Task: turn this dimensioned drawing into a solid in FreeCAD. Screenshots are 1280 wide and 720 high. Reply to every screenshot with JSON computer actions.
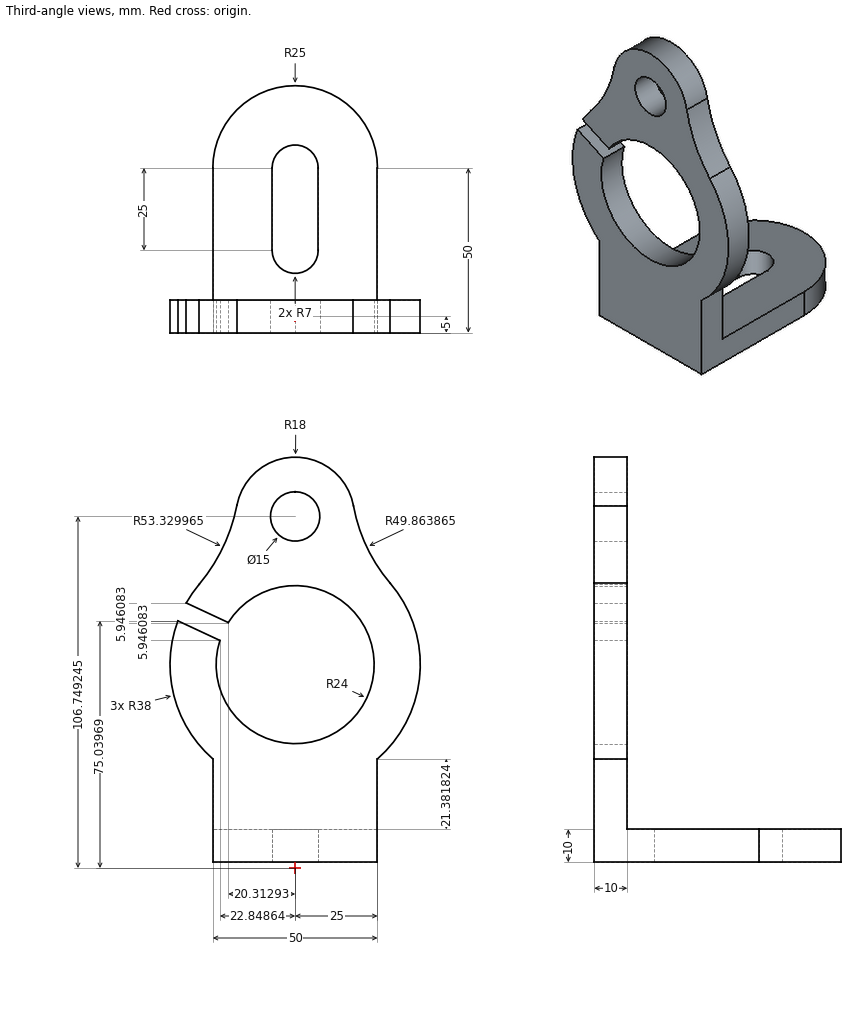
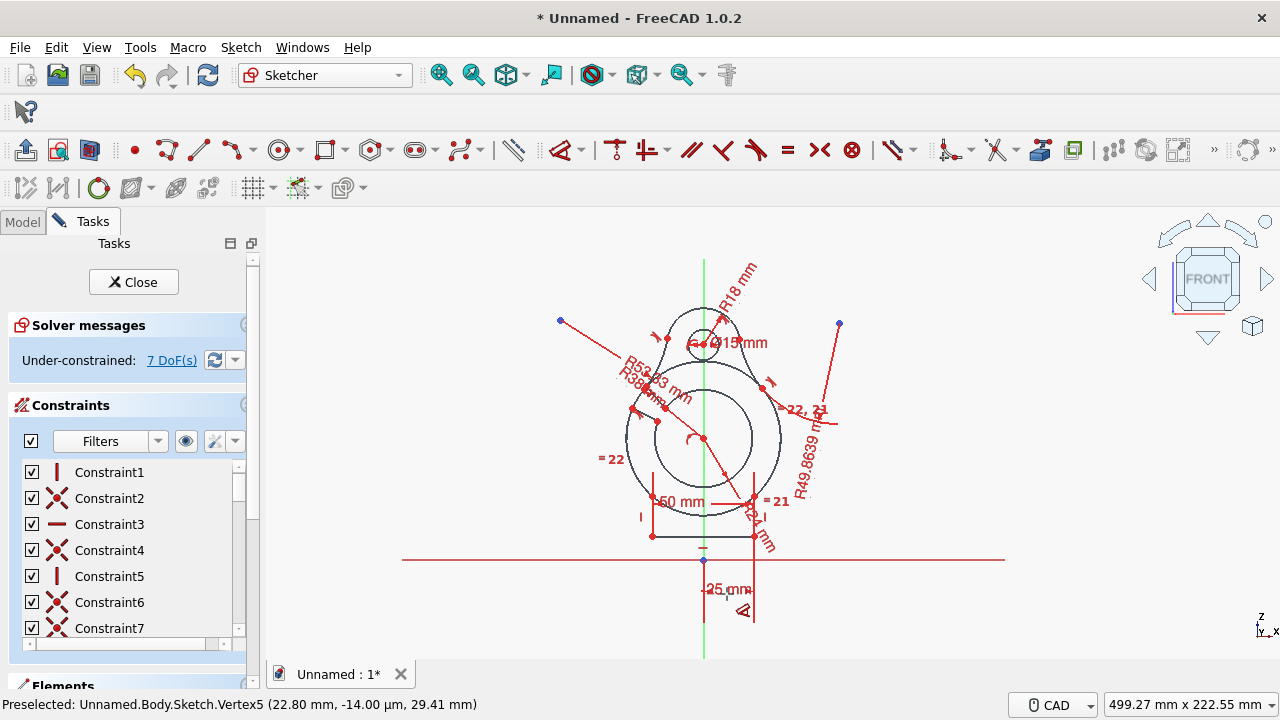
{"action": "scroll", "coordinate": [754, 509], "scroll_direction": "up", "scroll_amount": 2}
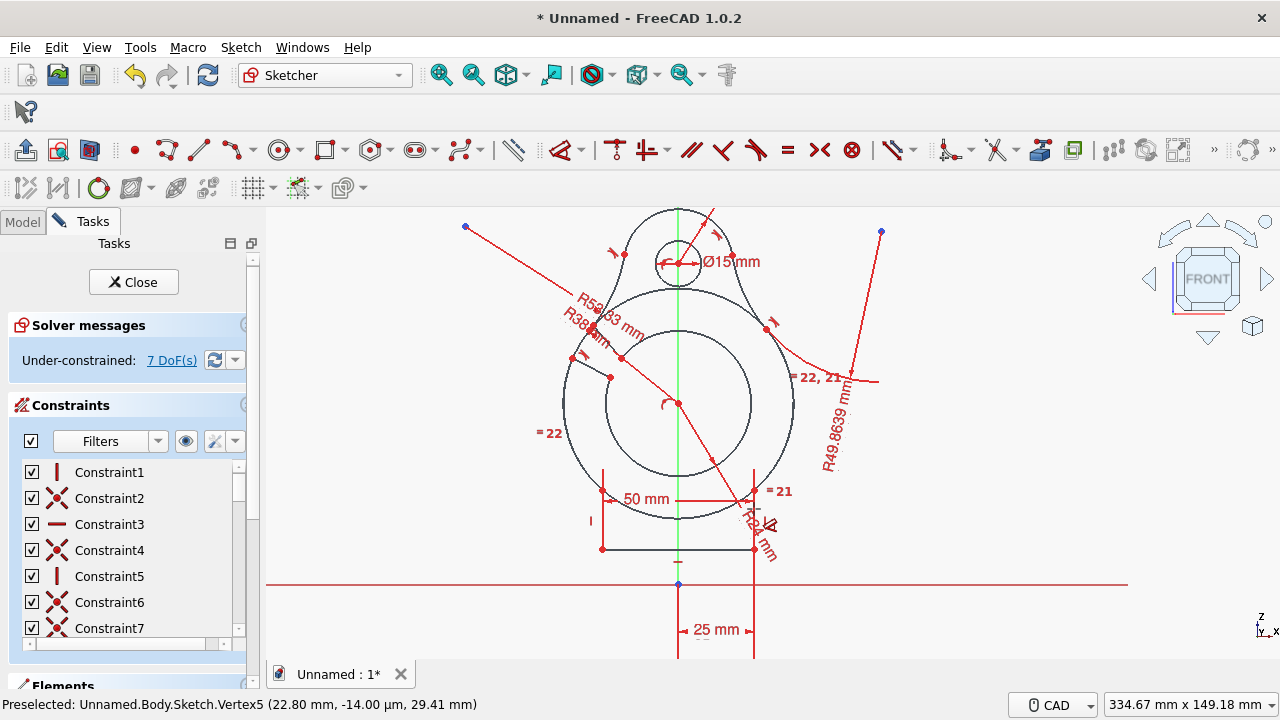
{"action": "left_click", "coordinate": [754, 508]}
{"action": "left_click", "coordinate": [788, 506]}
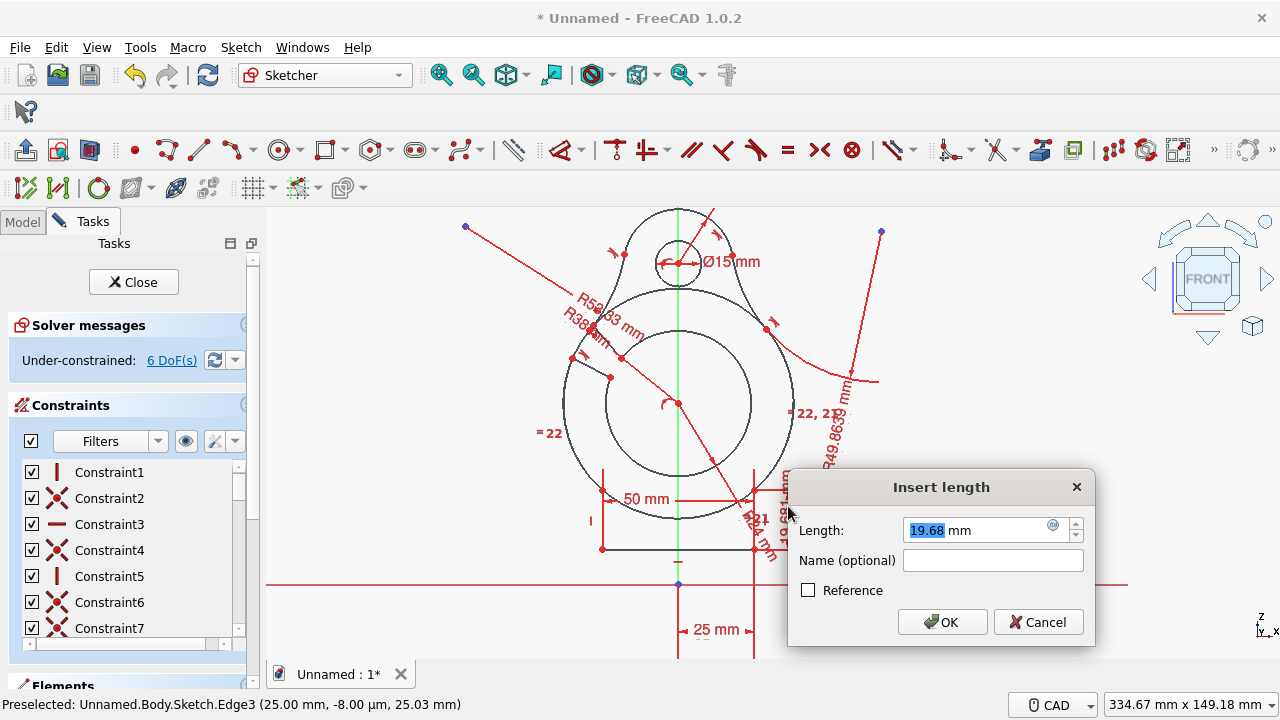
{"action": "type", "text": "21.381824"}
{"action": "key", "text": "Return"}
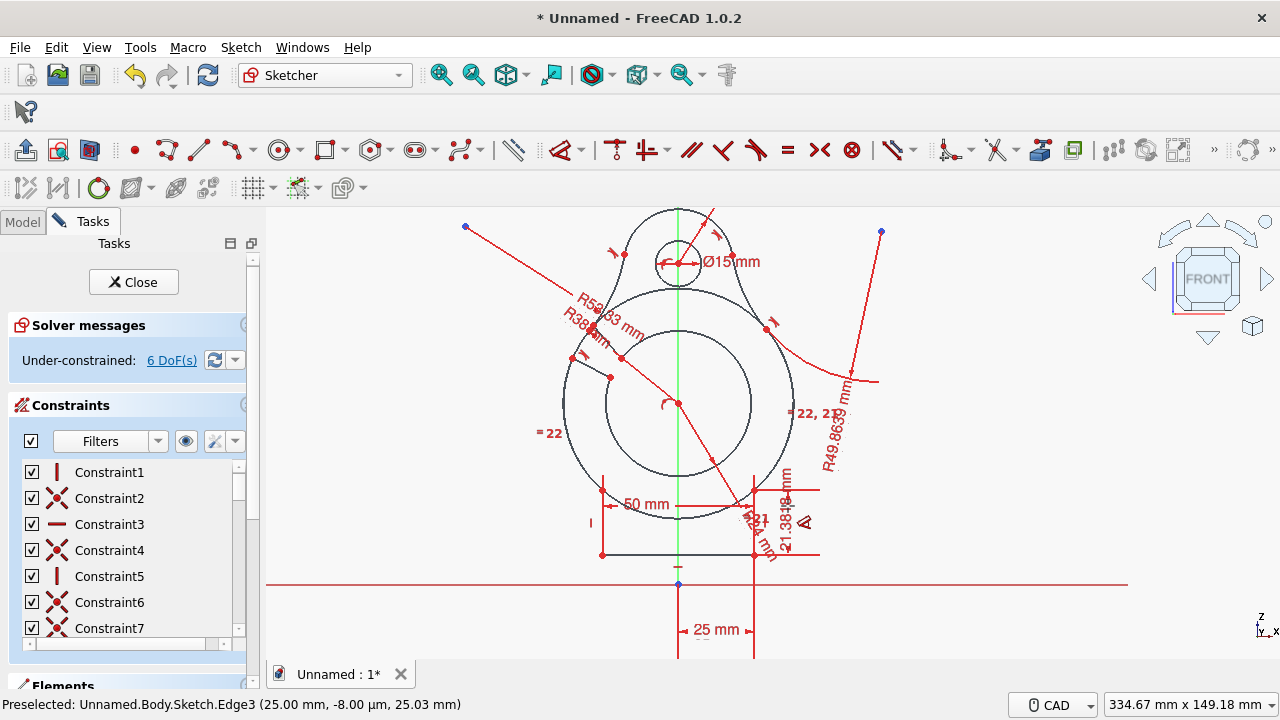
{"action": "left_click", "coordinate": [573, 358]}
{"action": "left_click", "coordinate": [539, 471]}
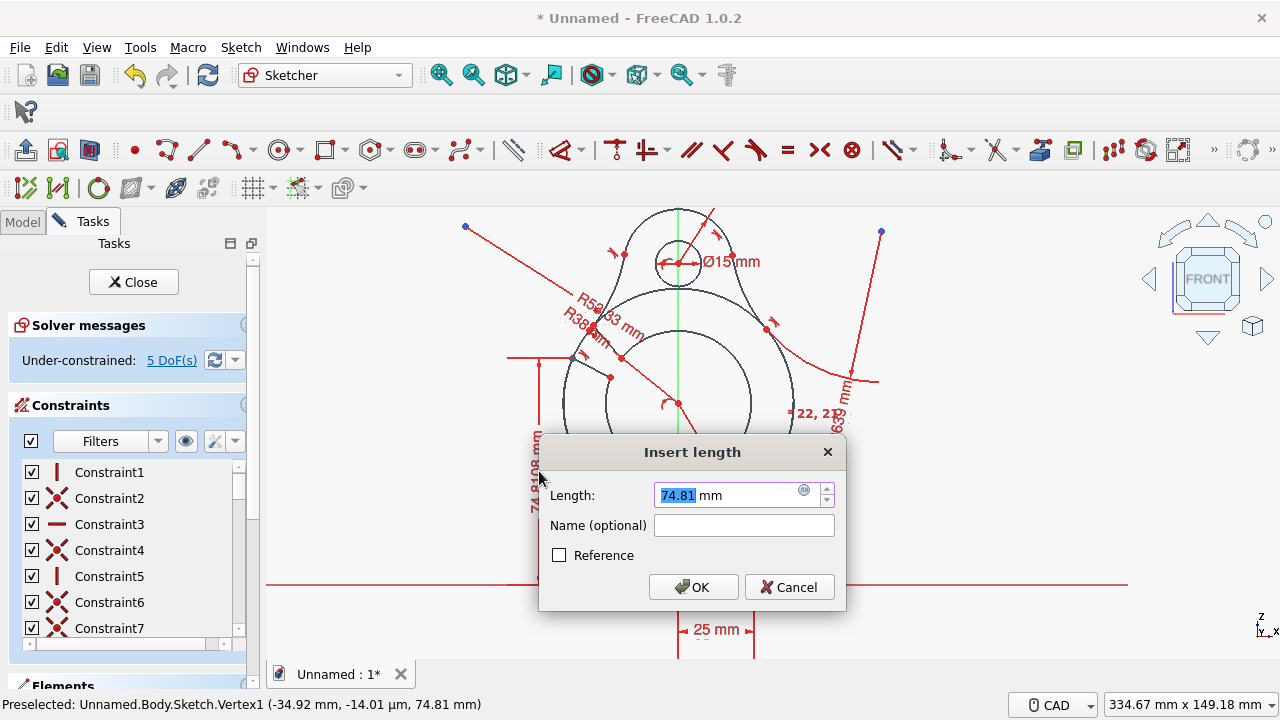
{"action": "type", "text": "75.03969"}
{"action": "key", "text": "Return"}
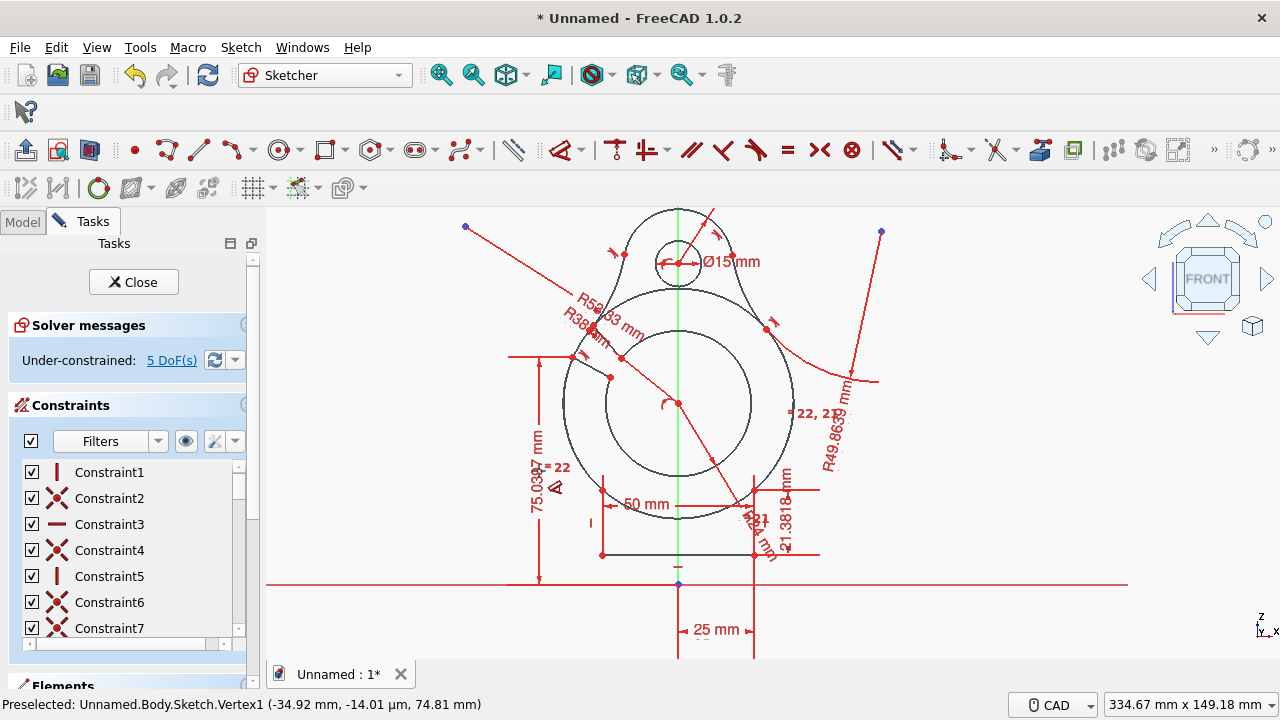
{"action": "left_click", "coordinate": [611, 378]}
{"action": "left_click", "coordinate": [629, 619]}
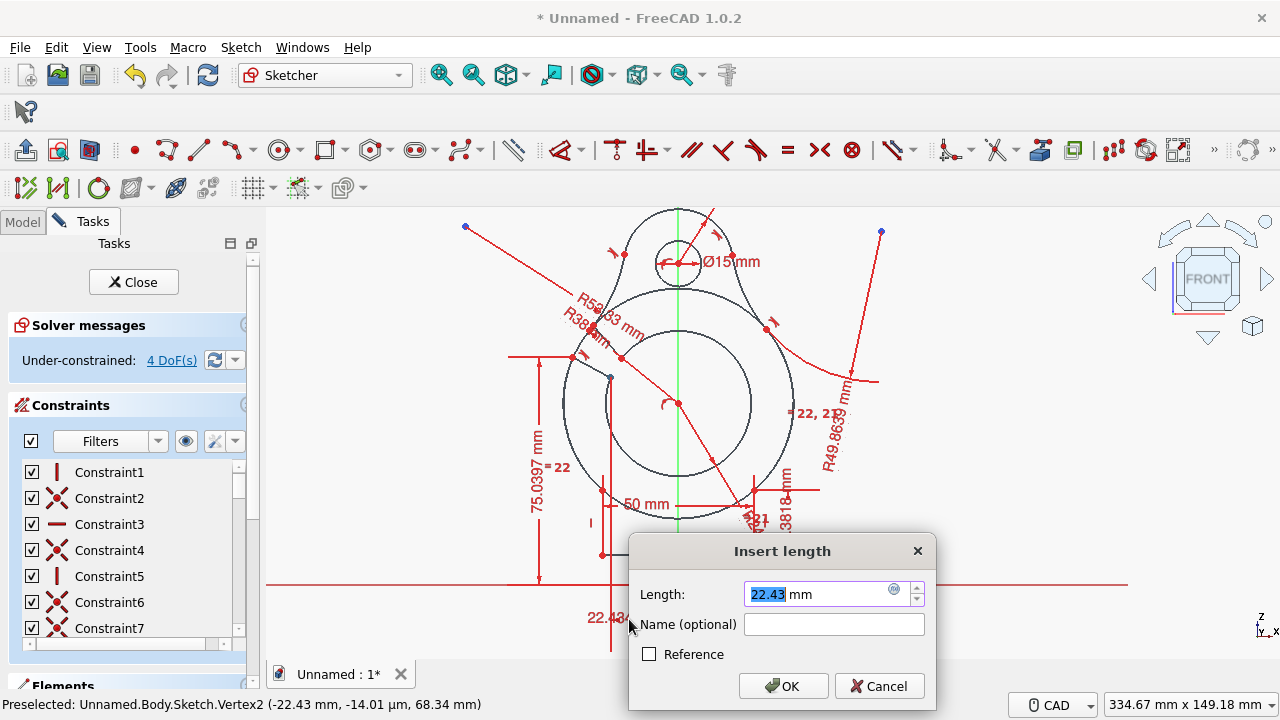
{"action": "type", "text": "22.84864"}
{"action": "key", "text": "Return"}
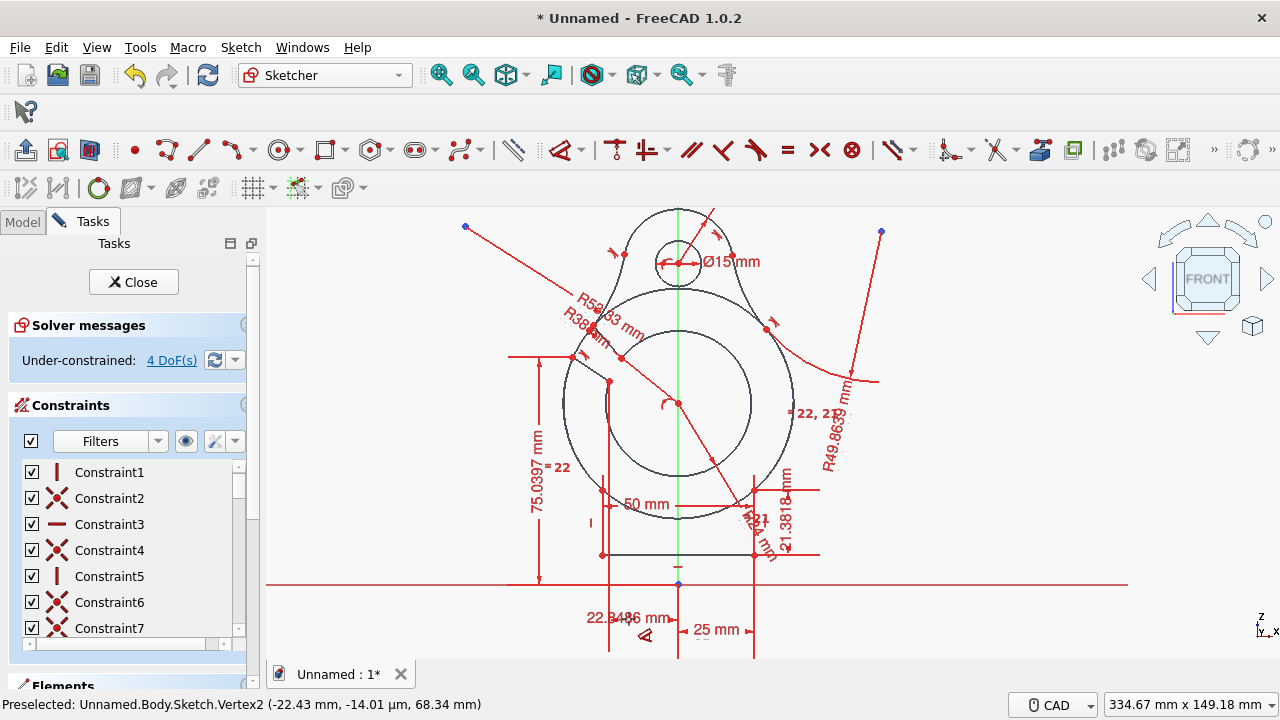
{"action": "left_click", "coordinate": [621, 359]}
{"action": "left_click", "coordinate": [637, 277]}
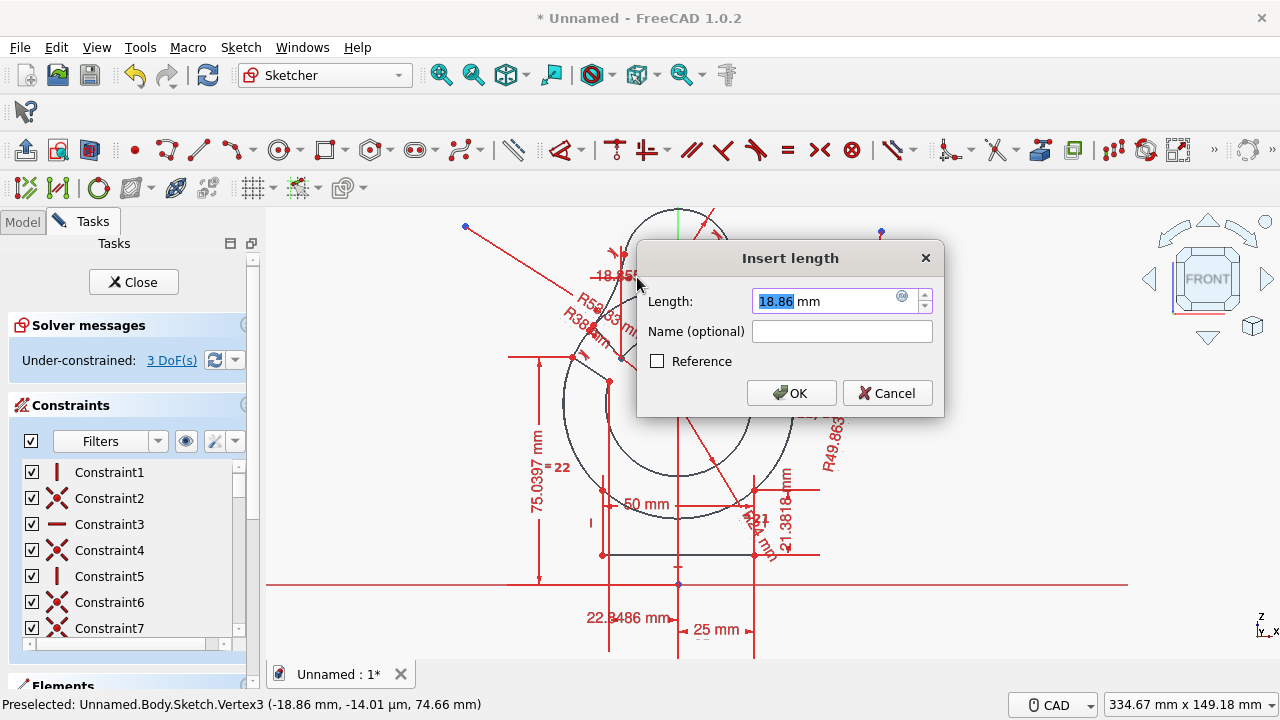
{"action": "type", "text": "20.31293"}
{"action": "key", "text": "Return"}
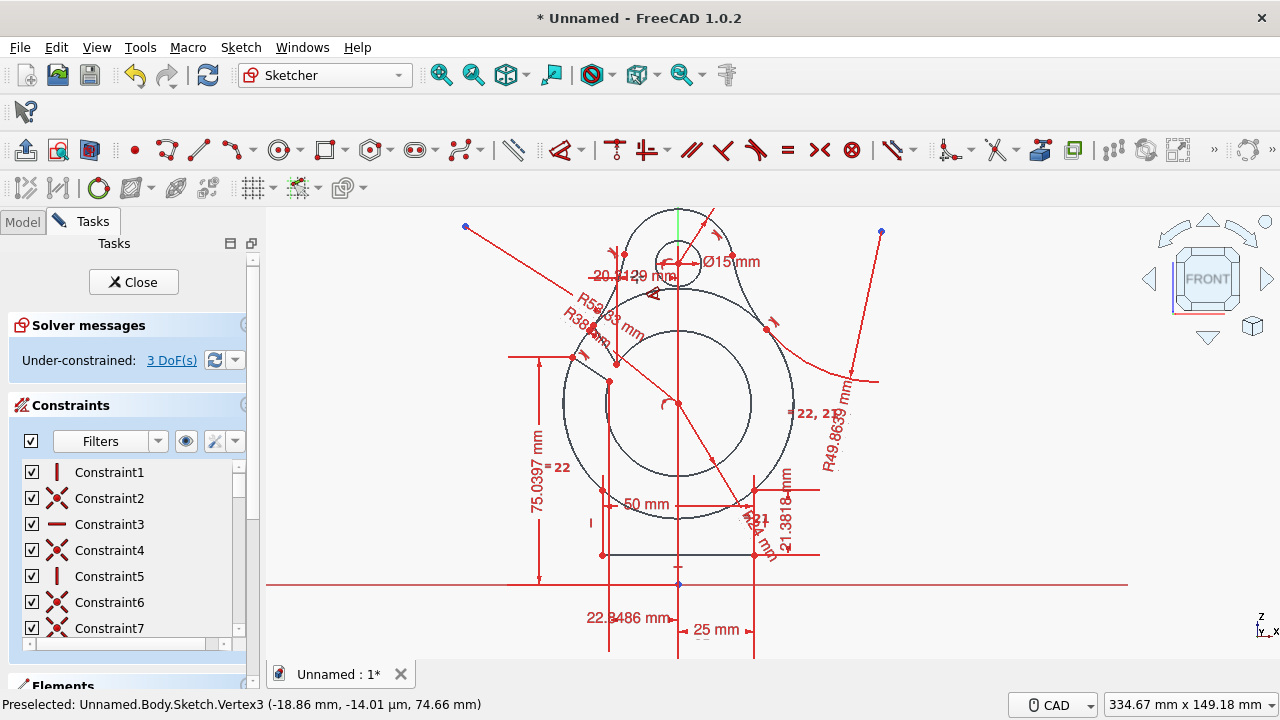
{"action": "scroll", "coordinate": [584, 365], "scroll_direction": "up", "scroll_amount": 4}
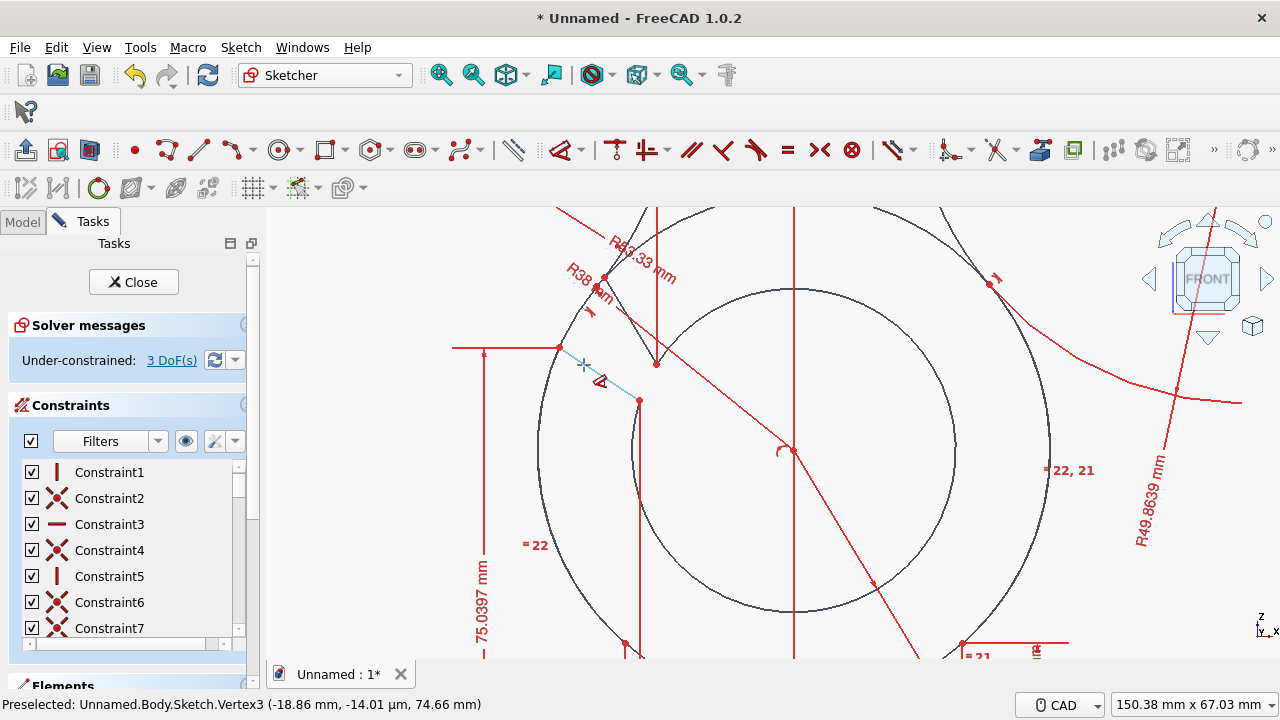
{"action": "left_click", "coordinate": [583, 364]}
{"action": "left_click", "coordinate": [525, 374]}